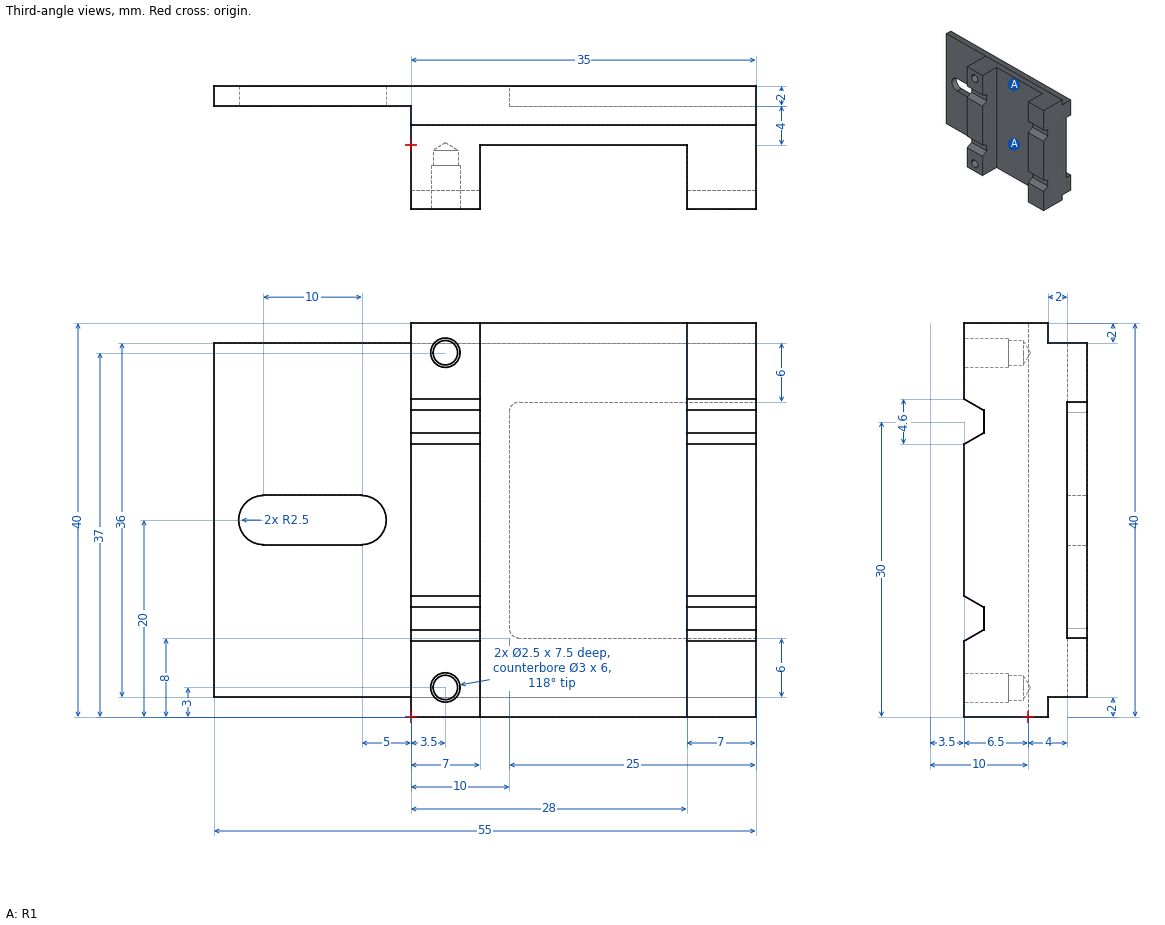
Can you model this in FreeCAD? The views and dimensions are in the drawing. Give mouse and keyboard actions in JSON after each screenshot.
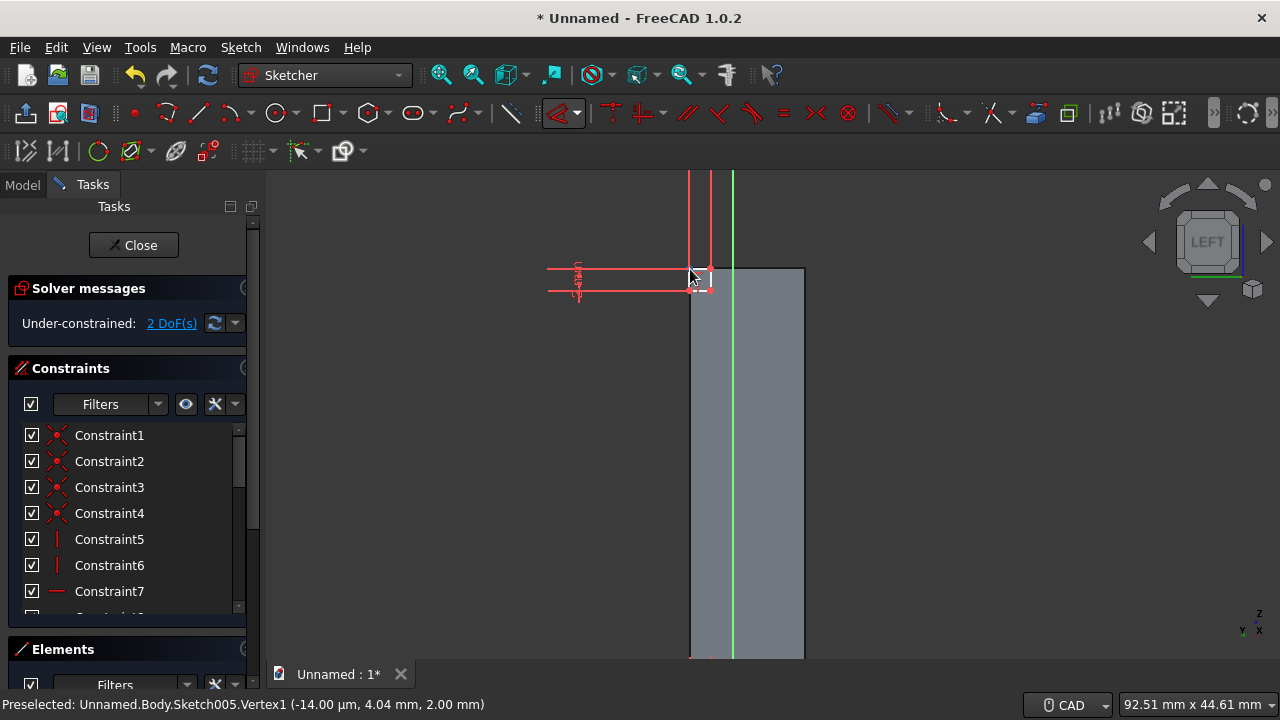
{"action": "left_click", "coordinate": [689, 269]}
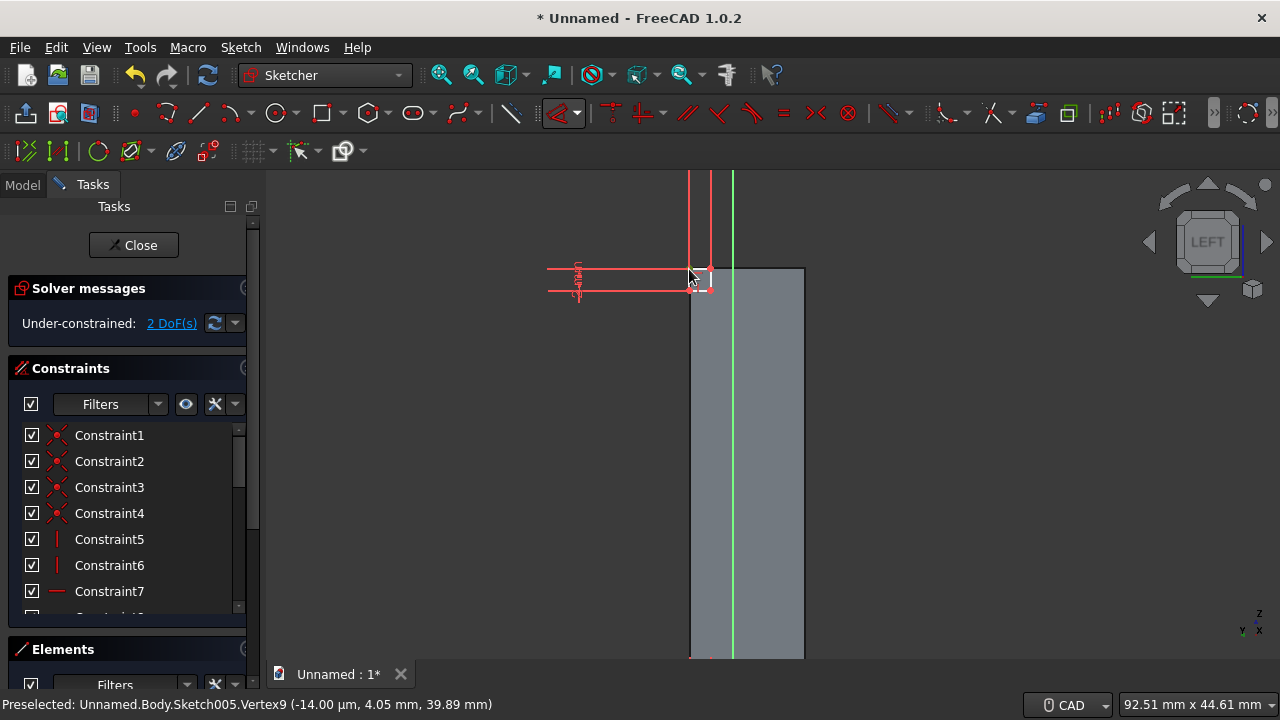
{"action": "left_click", "coordinate": [580, 114]}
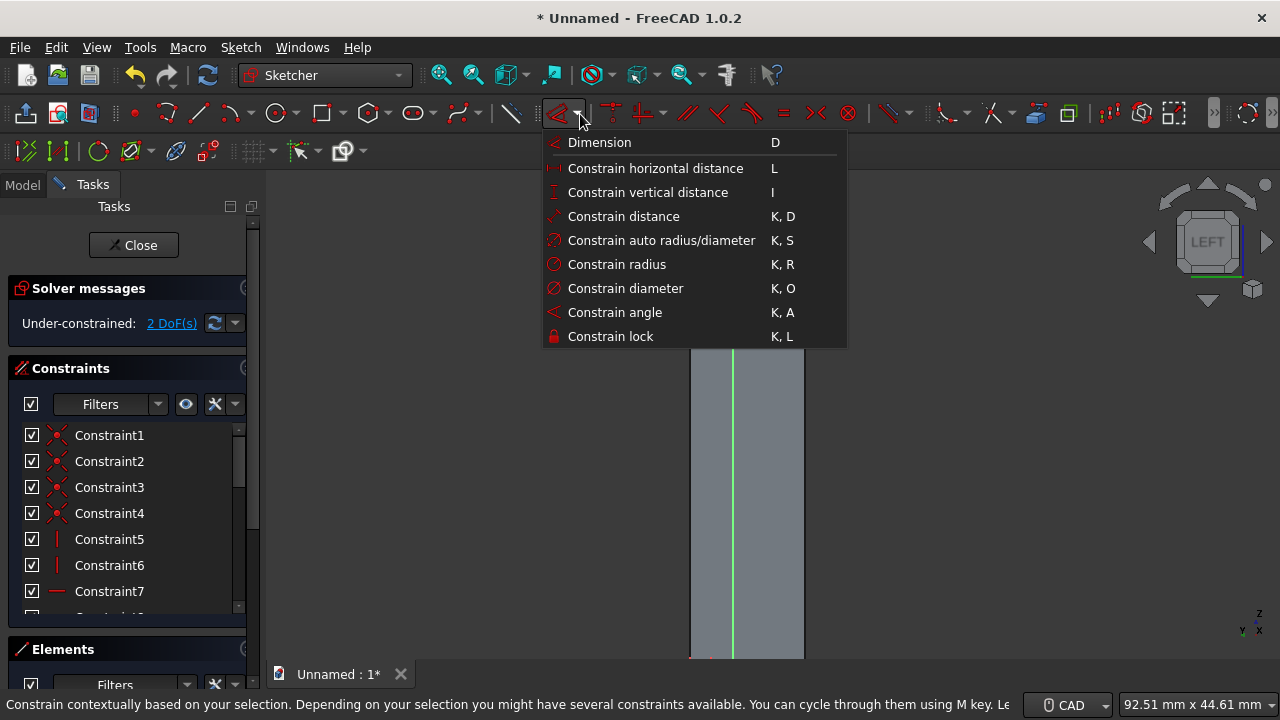
{"action": "left_click", "coordinate": [695, 168]}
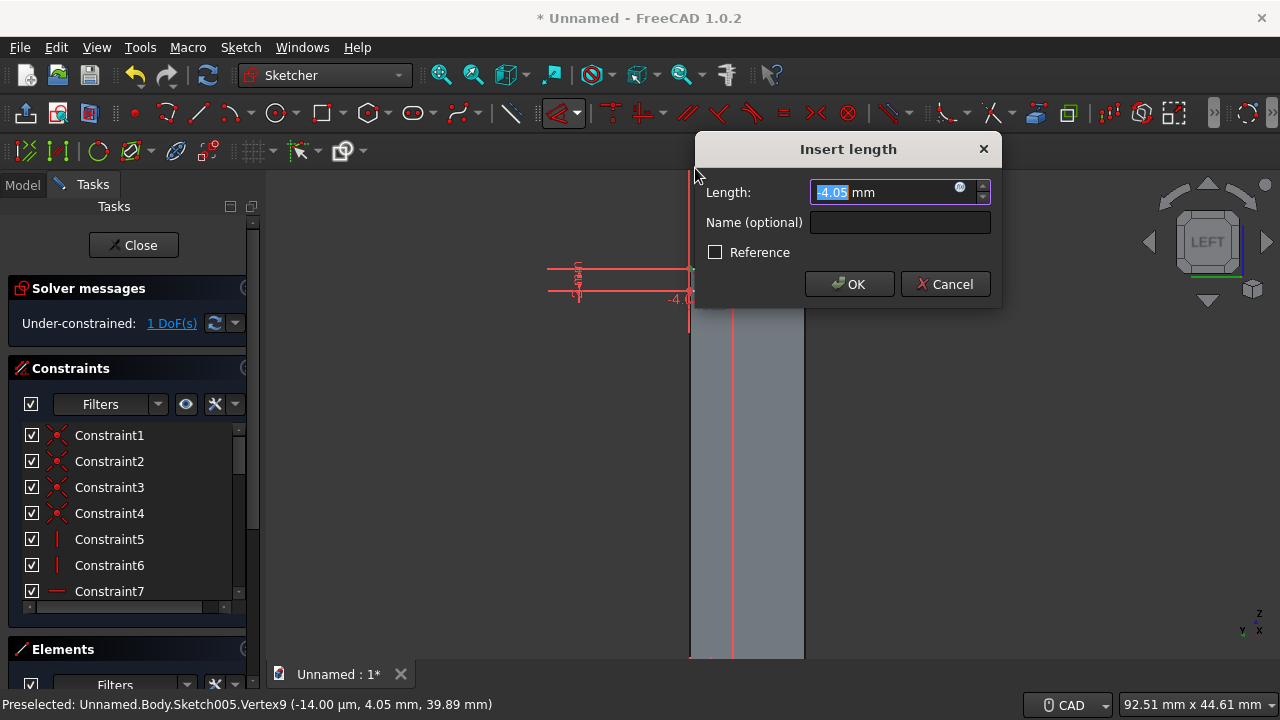
{"action": "type", "text": "-4"}
{"action": "key", "text": "Return"}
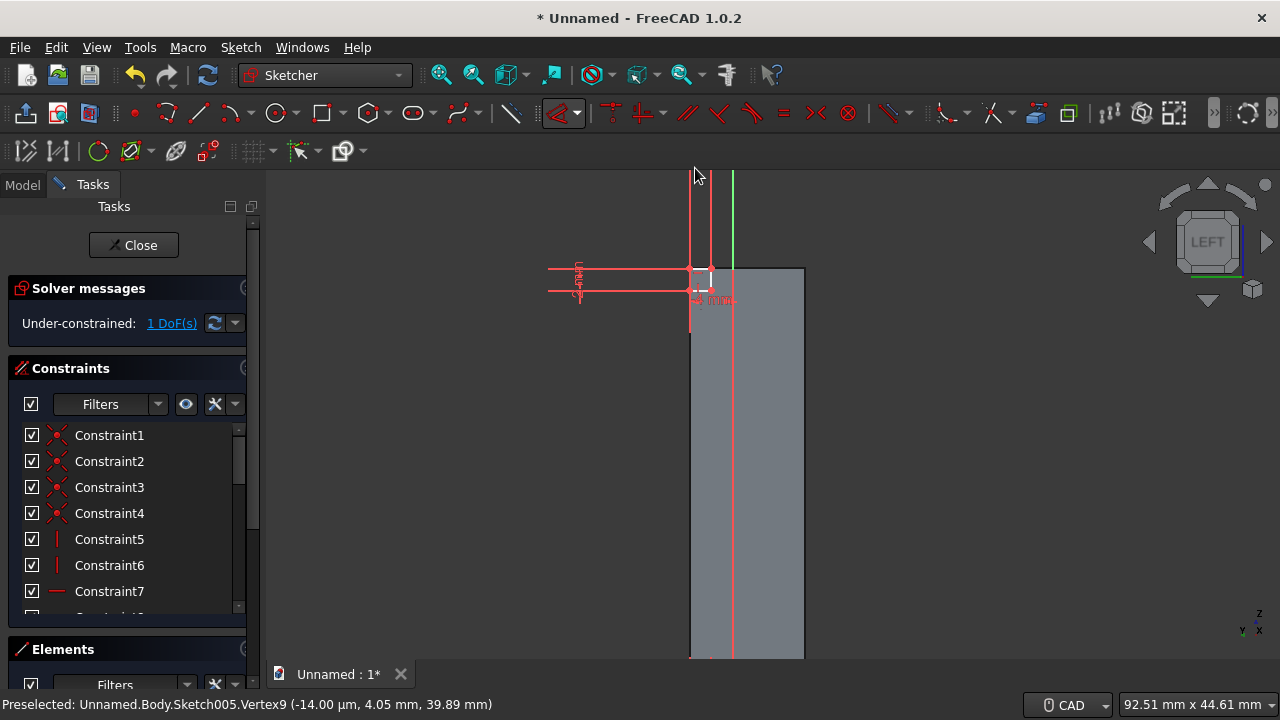
{"action": "left_click", "coordinate": [690, 269]}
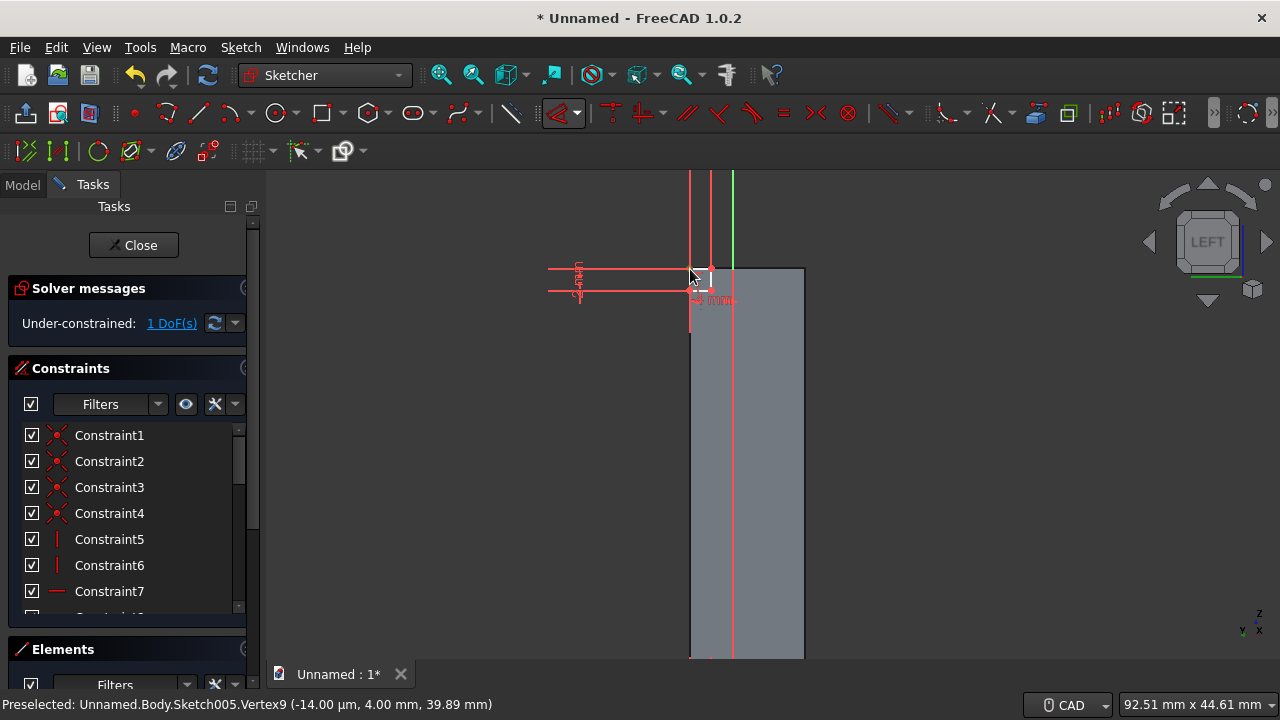
{"action": "left_click", "coordinate": [580, 114]}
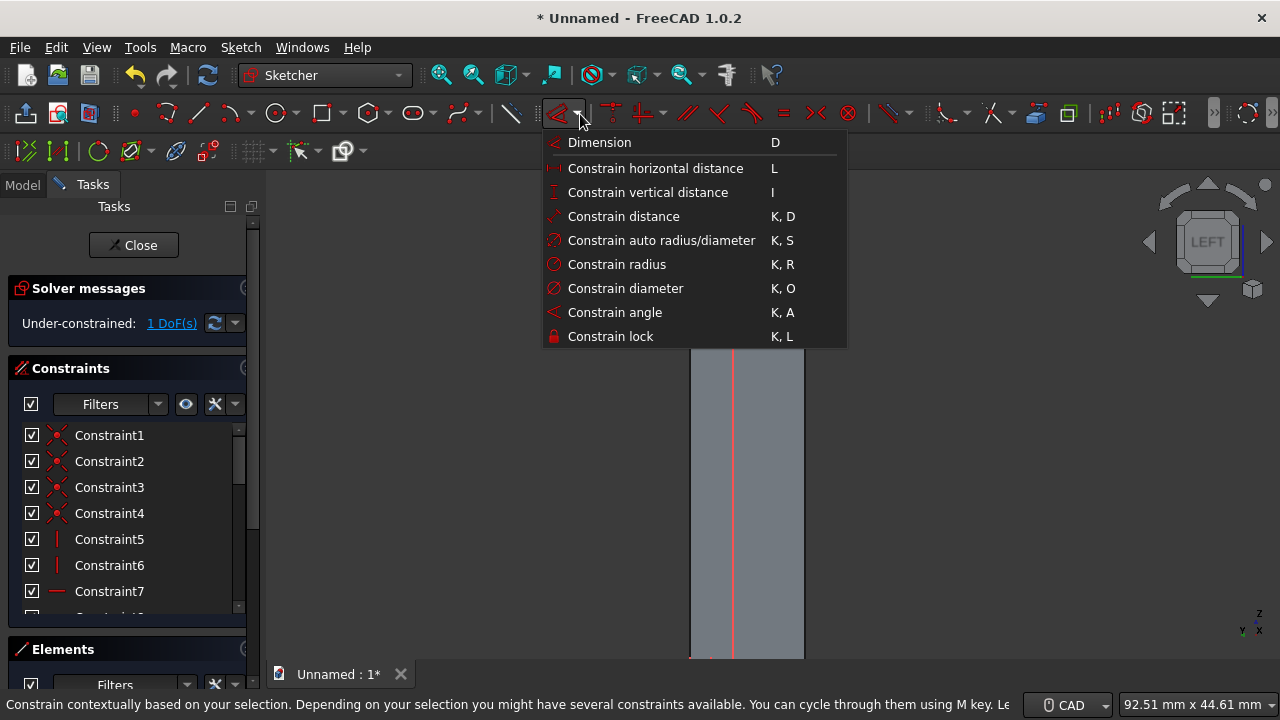
{"action": "left_click", "coordinate": [695, 192]}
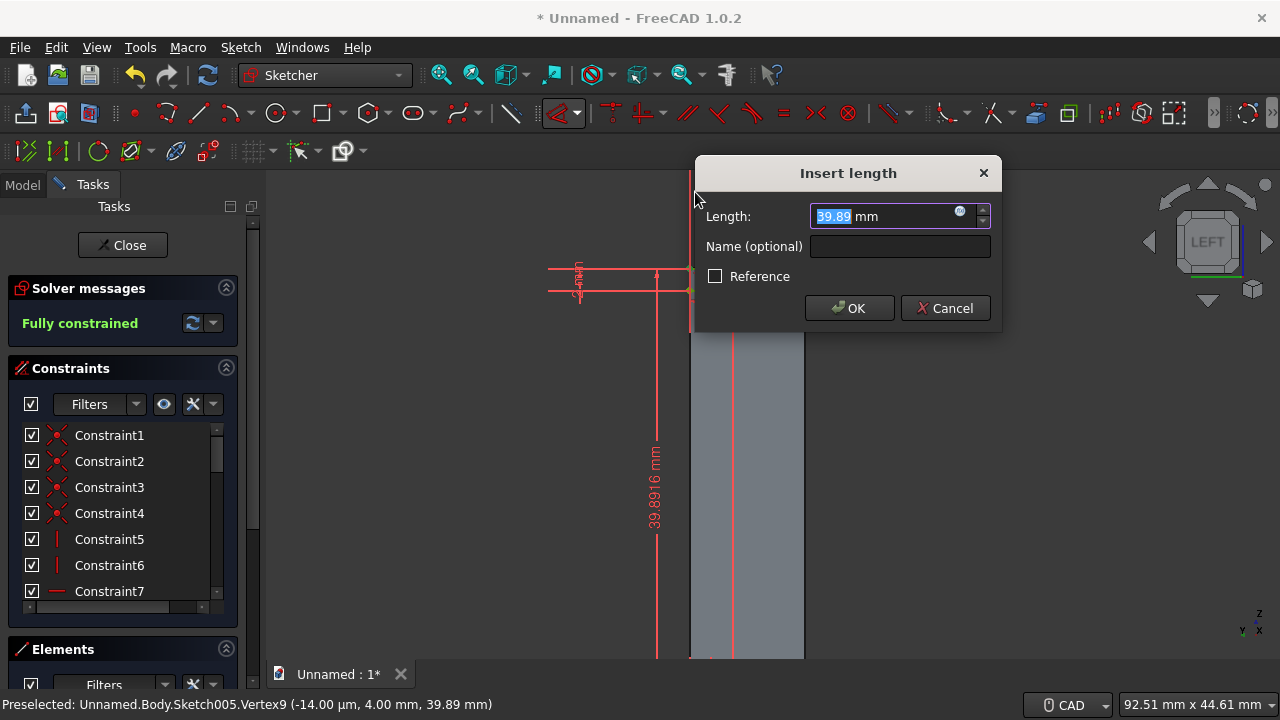
{"action": "type", "text": "40"}
{"action": "key", "text": "Return"}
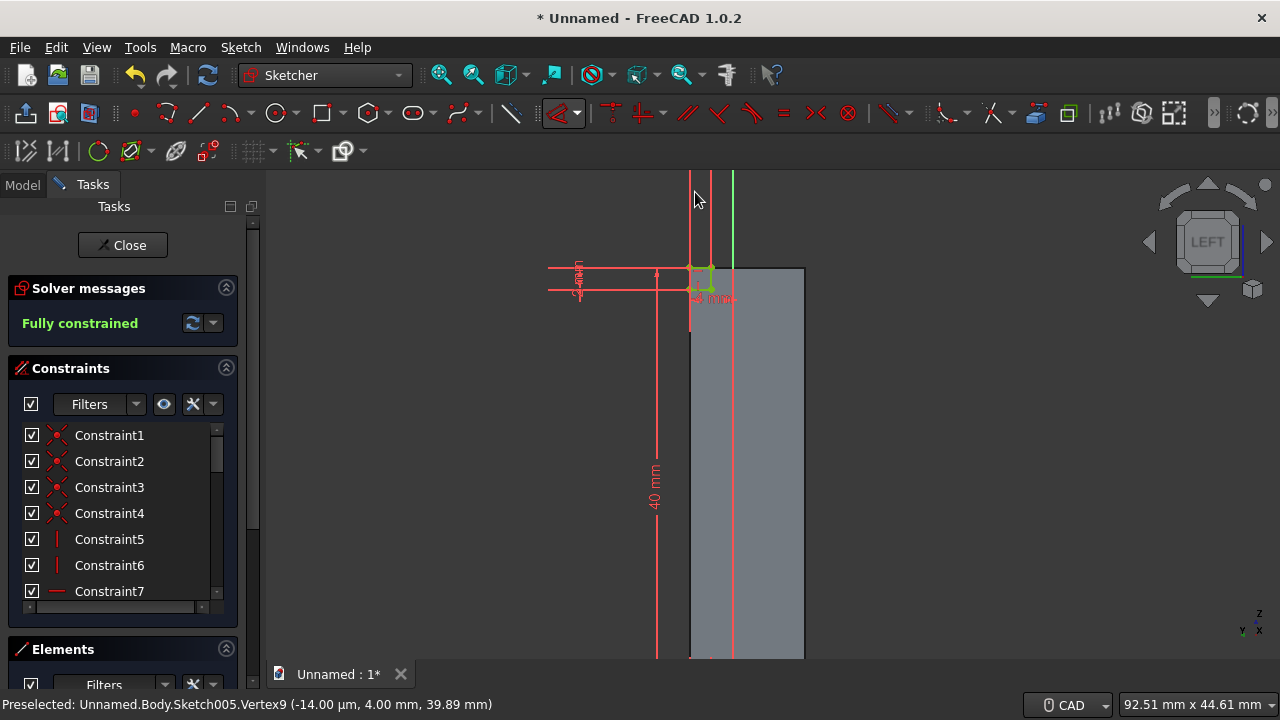
{"action": "left_click", "coordinate": [123, 245]}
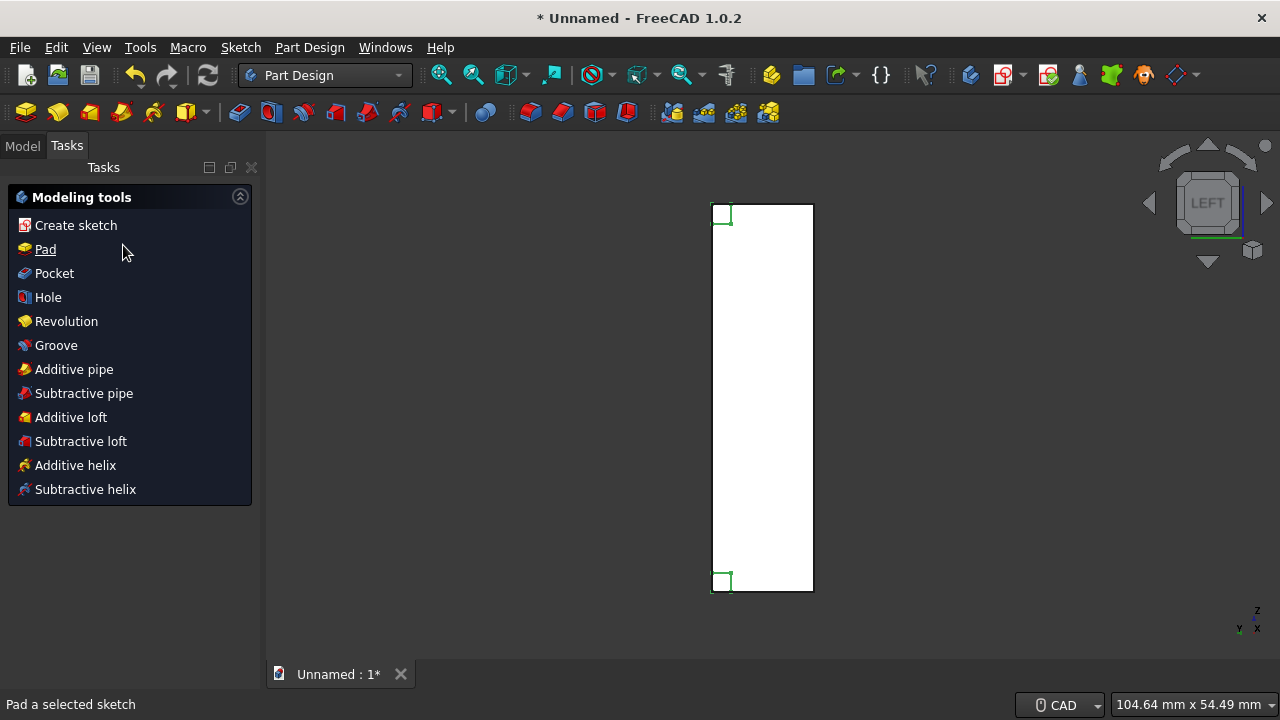
{"action": "left_click", "coordinate": [240, 112]}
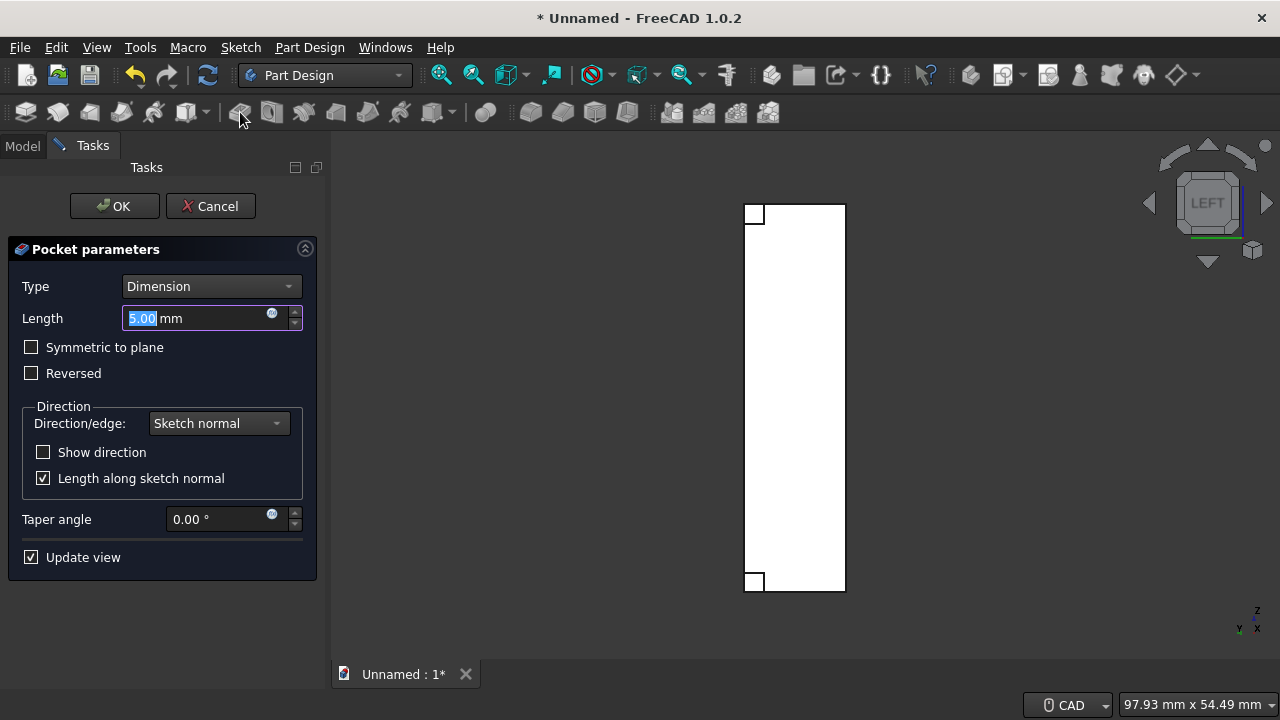
{"action": "left_click", "coordinate": [212, 286]}